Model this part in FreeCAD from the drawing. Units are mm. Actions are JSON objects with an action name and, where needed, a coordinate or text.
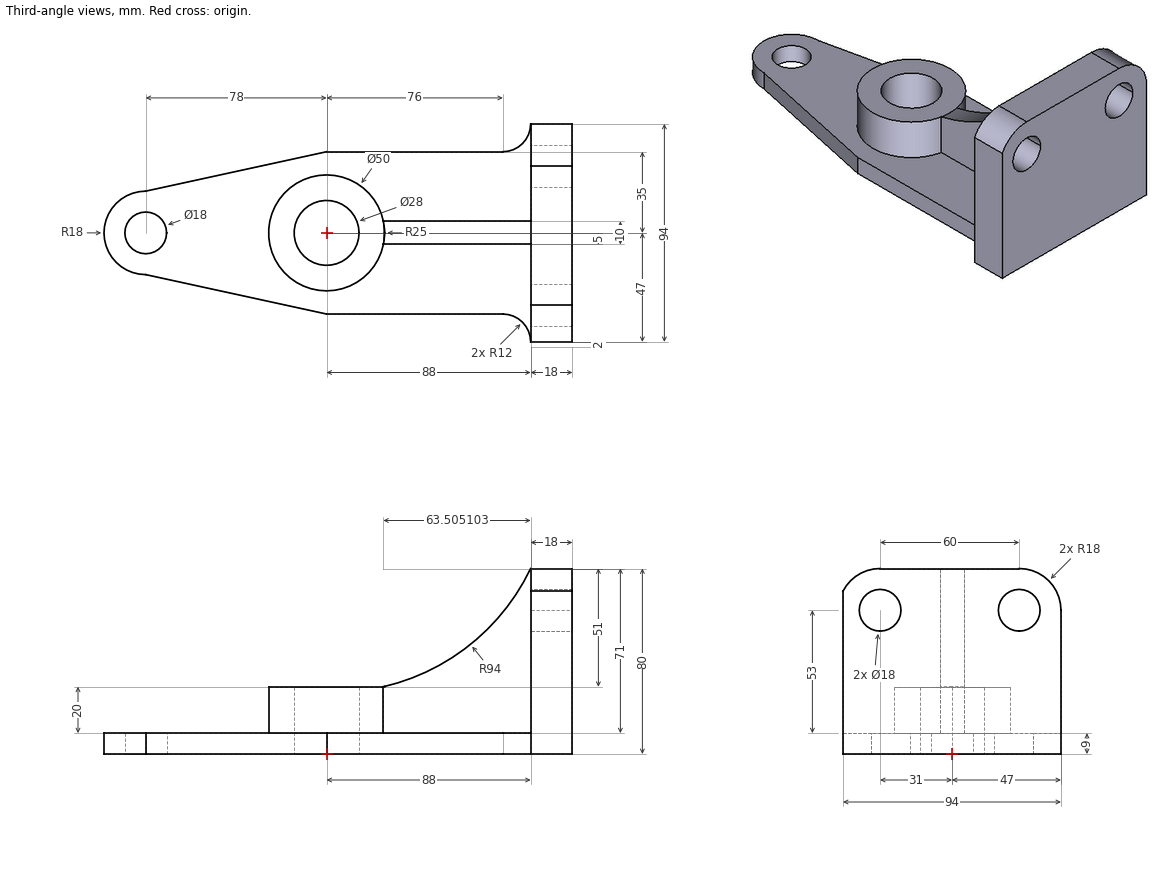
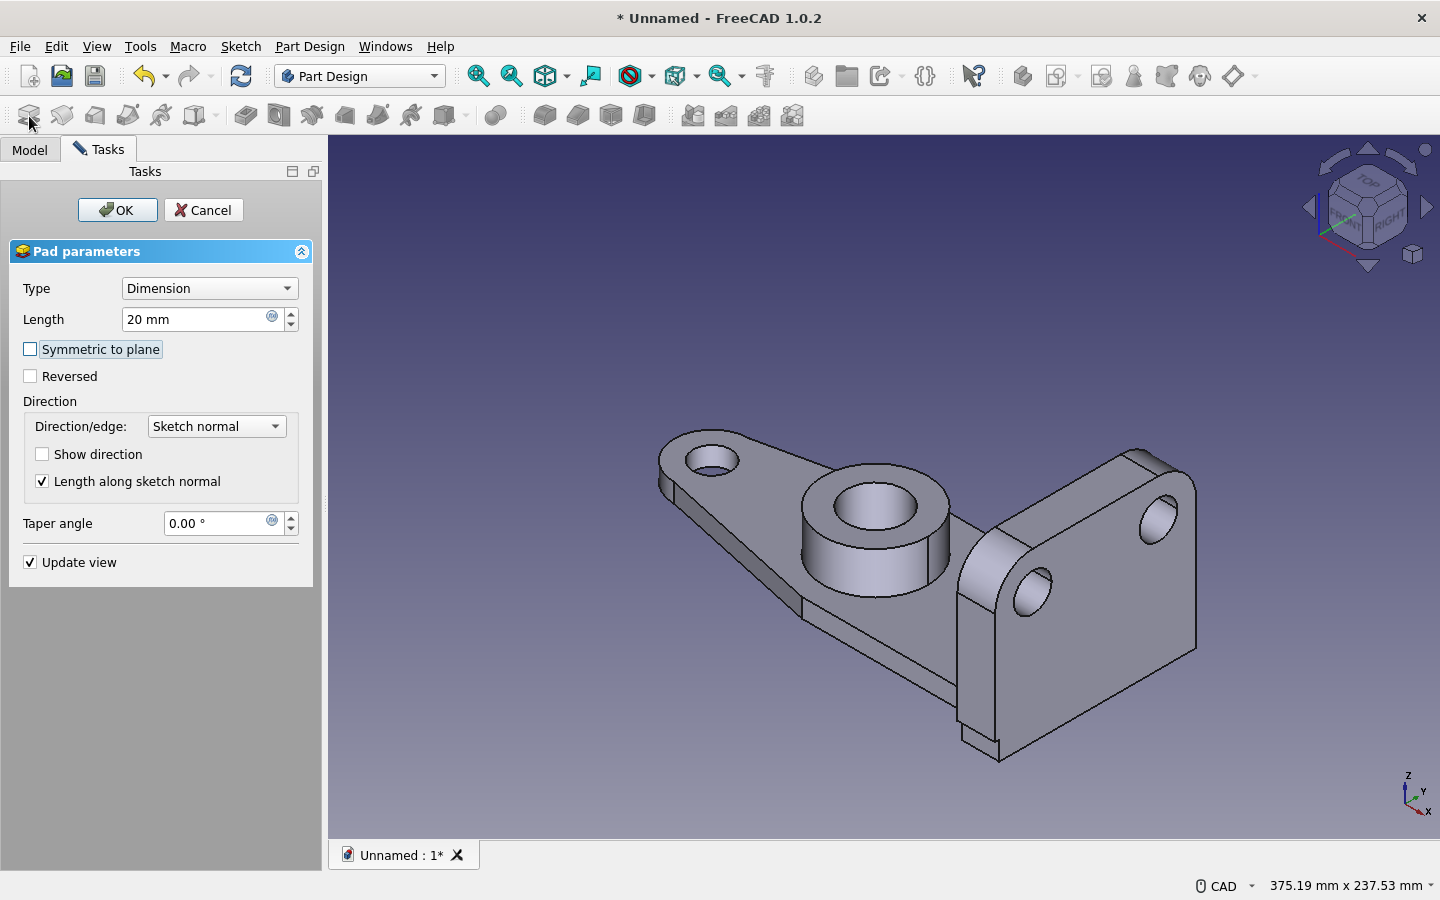
{"action": "left_click", "coordinate": [118, 210]}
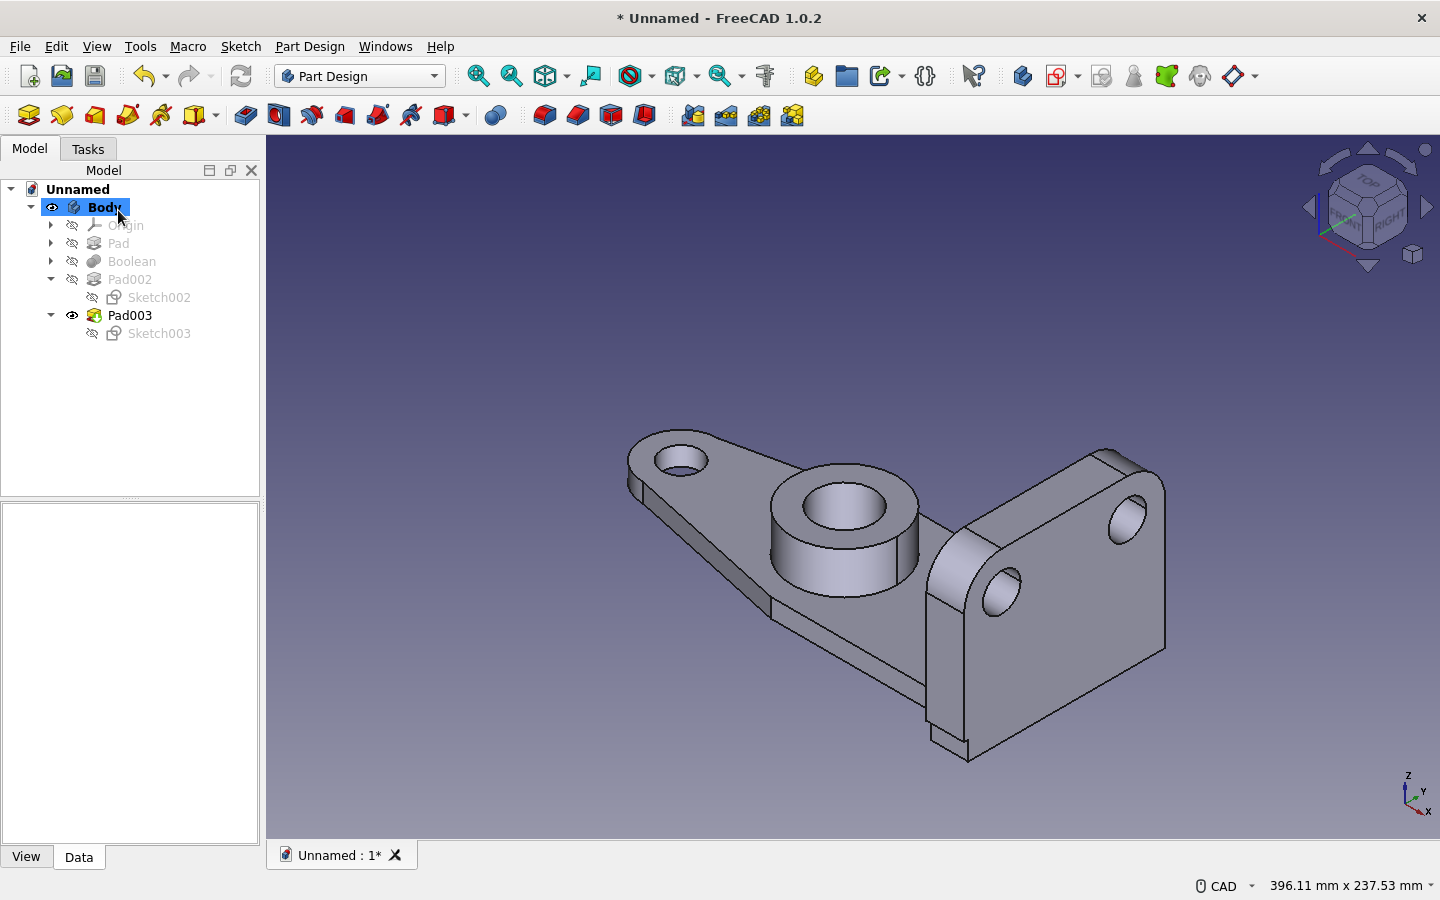
{"action": "left_click", "coordinate": [918, 629]}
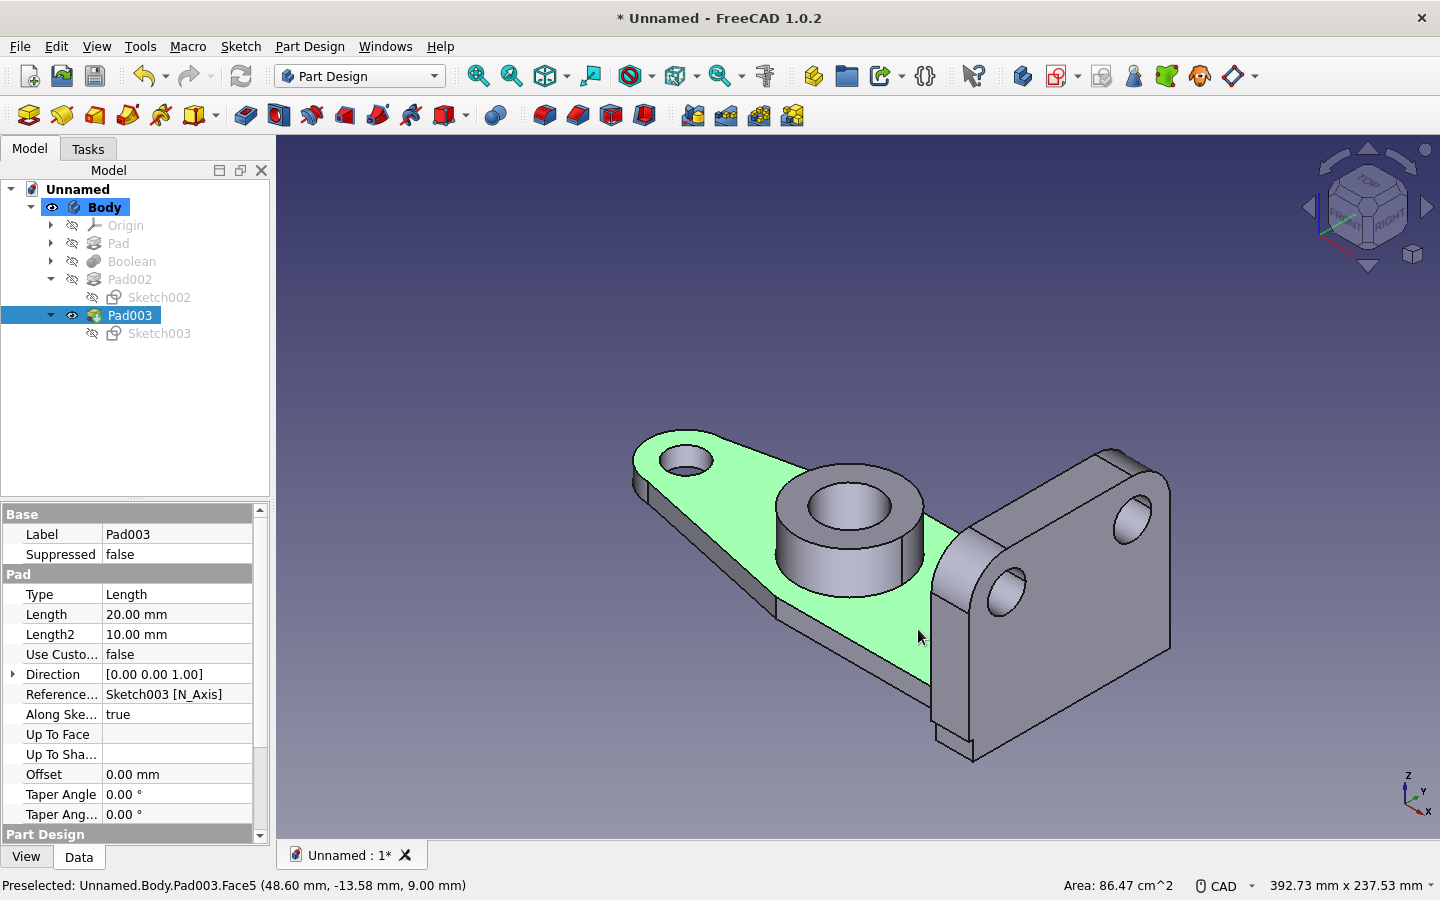
{"action": "left_click", "coordinate": [1056, 76]}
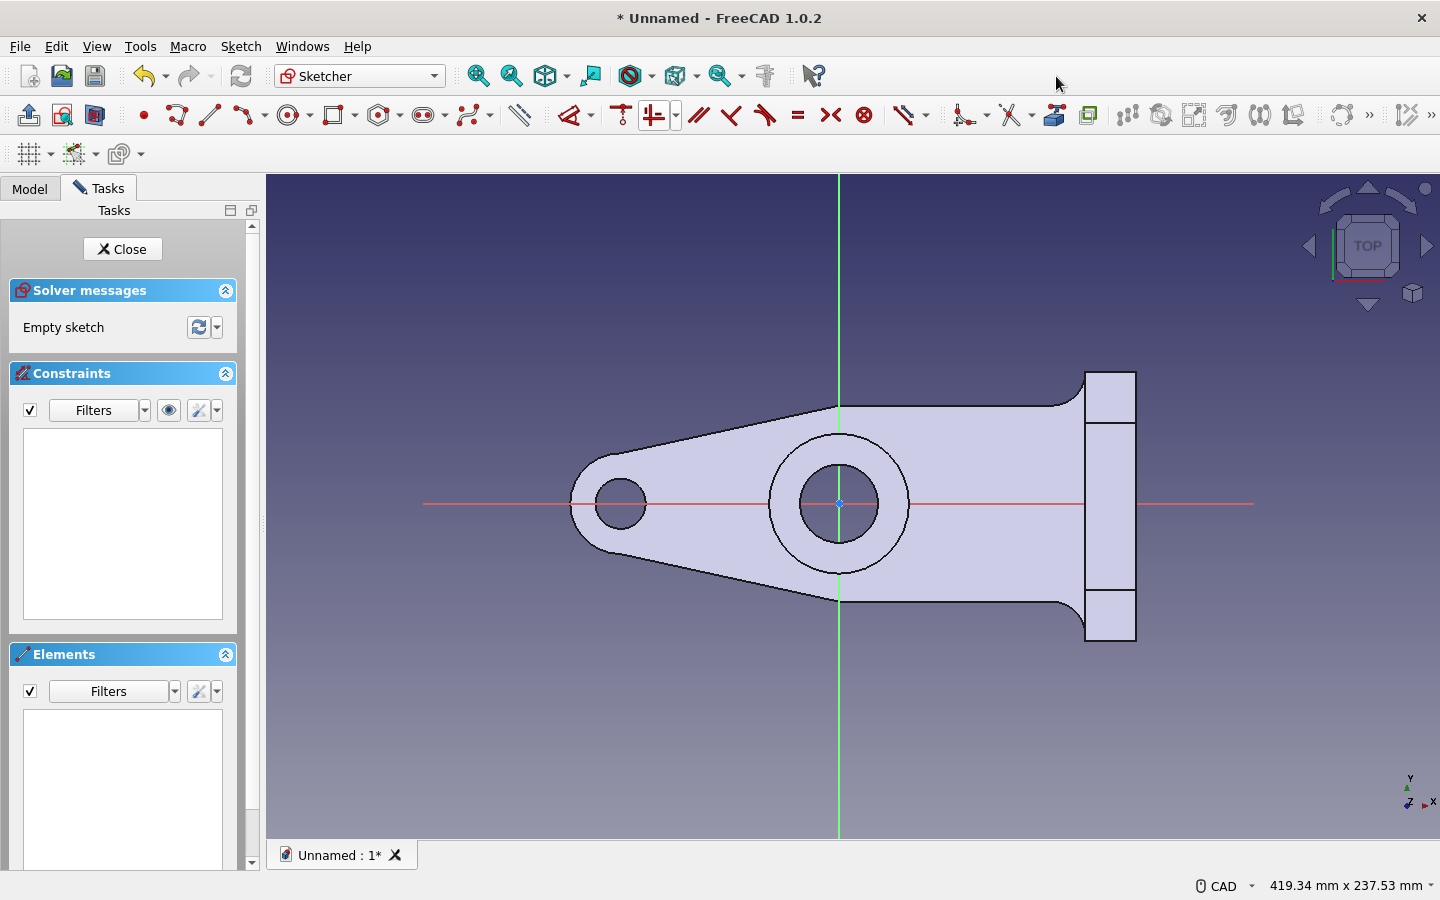
{"action": "scroll", "coordinate": [1066, 502], "scroll_direction": "up", "scroll_amount": 5}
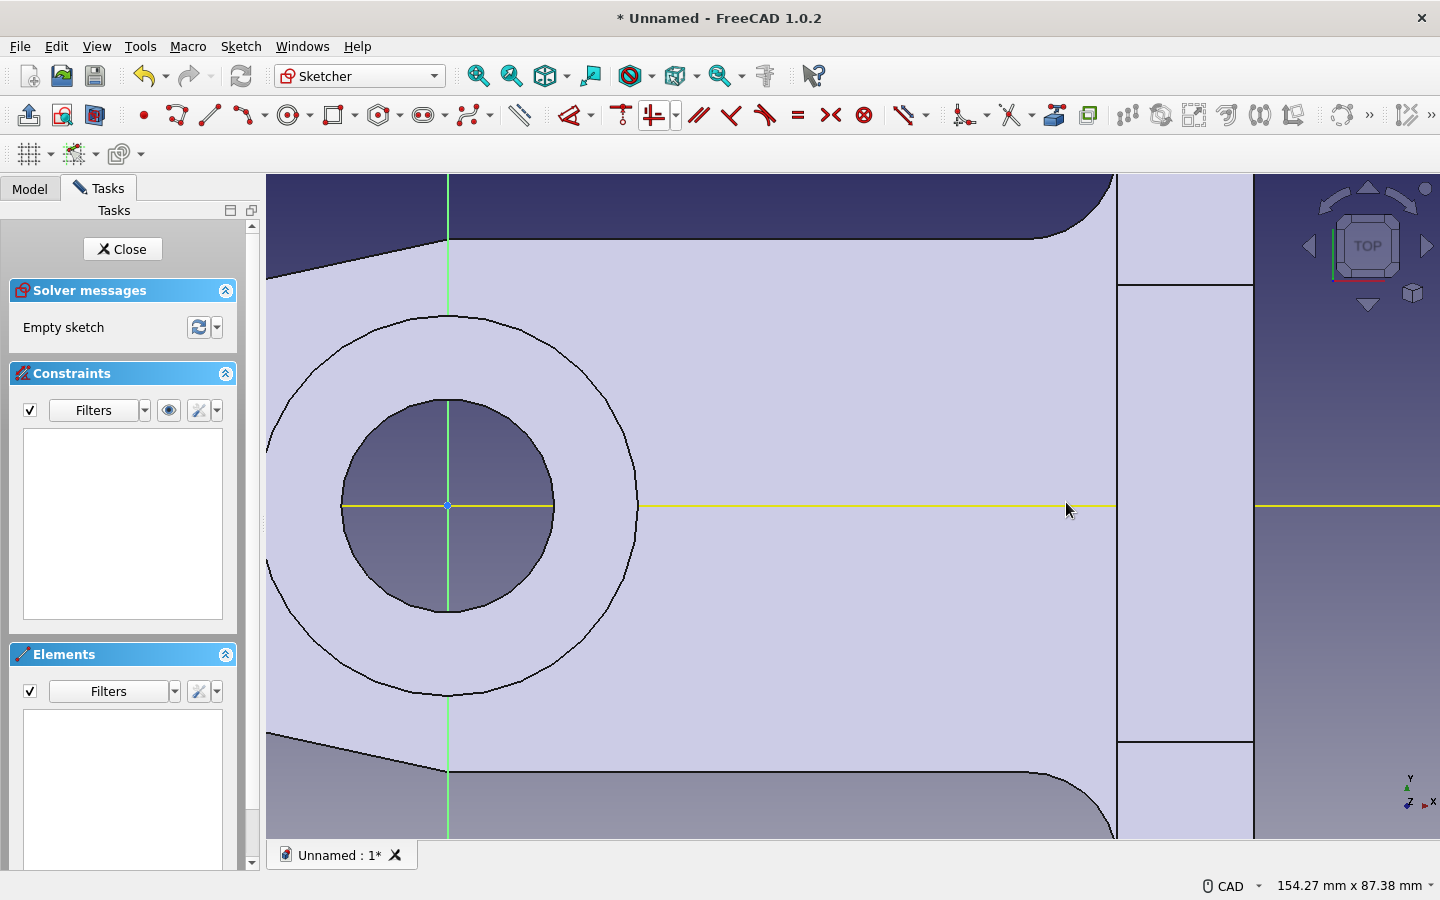
{"action": "left_click", "coordinate": [177, 116]}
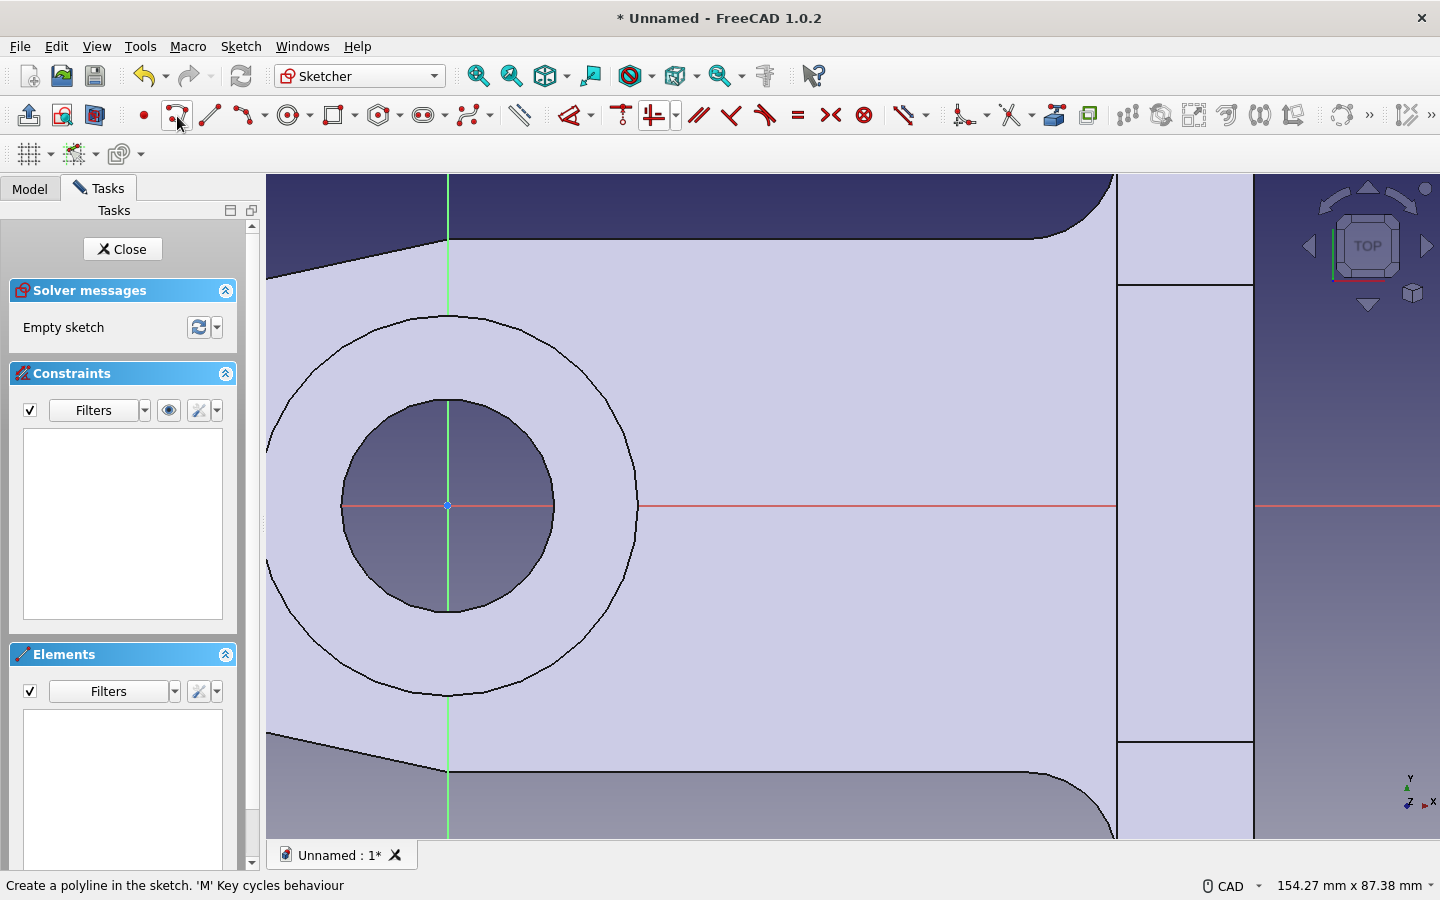
{"action": "left_click", "coordinate": [634, 544]}
{"action": "left_click", "coordinate": [1117, 544]}
{"action": "left_click", "coordinate": [1117, 468]}
{"action": "left_click", "coordinate": [634, 468]}
{"action": "right_click", "coordinate": [634, 468]}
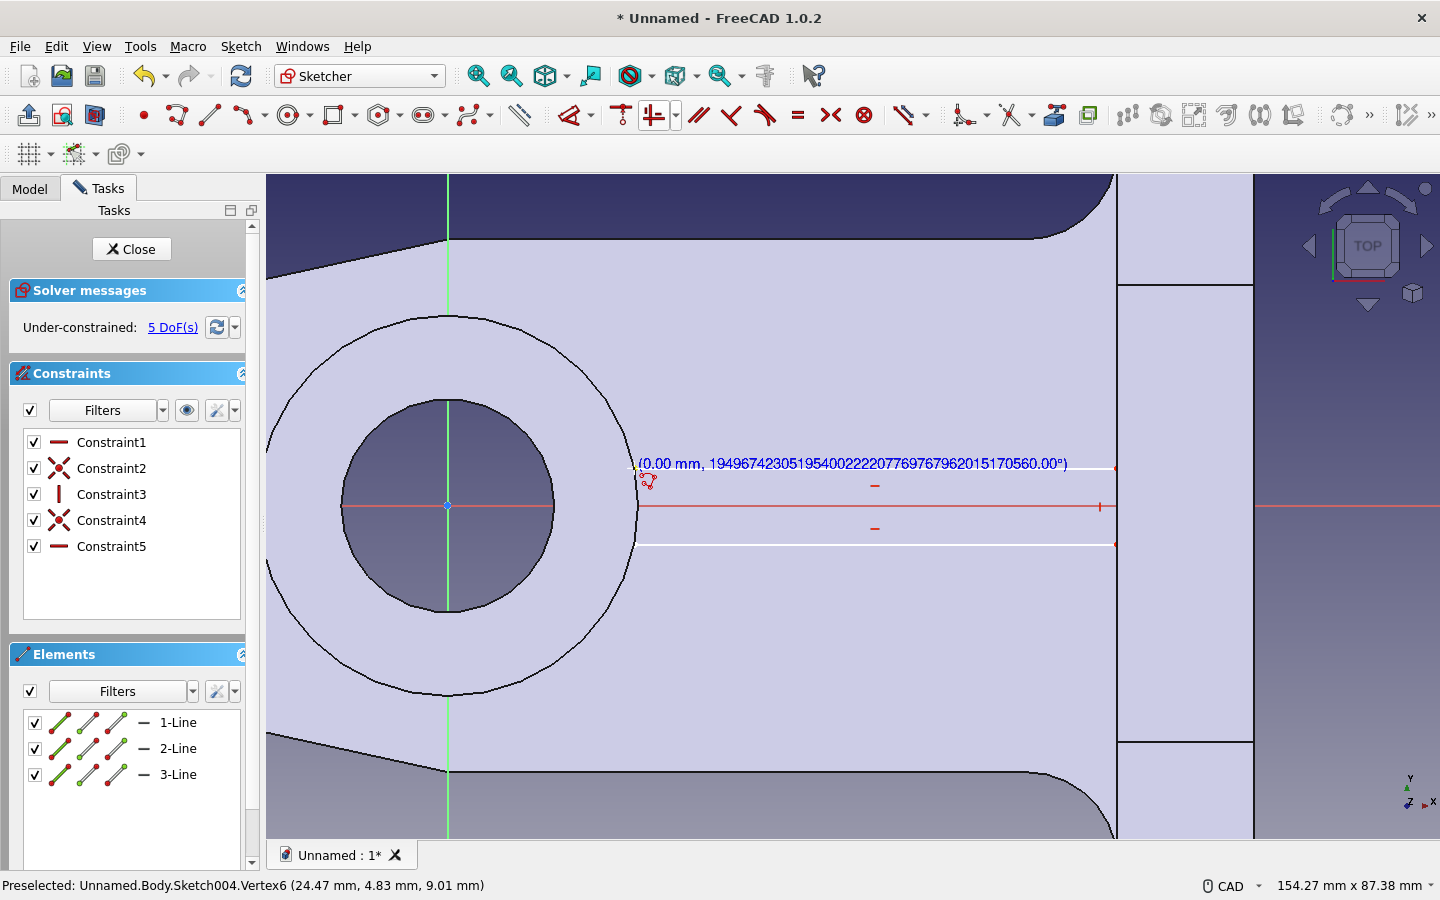
{"action": "left_click", "coordinate": [242, 116]}